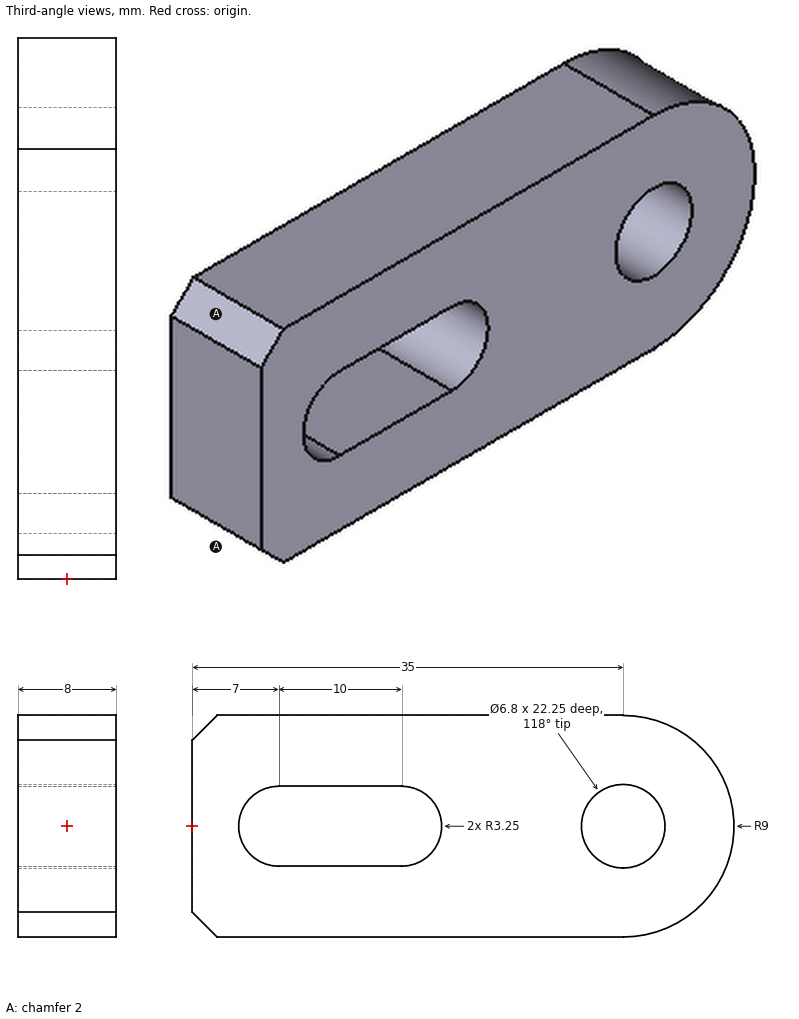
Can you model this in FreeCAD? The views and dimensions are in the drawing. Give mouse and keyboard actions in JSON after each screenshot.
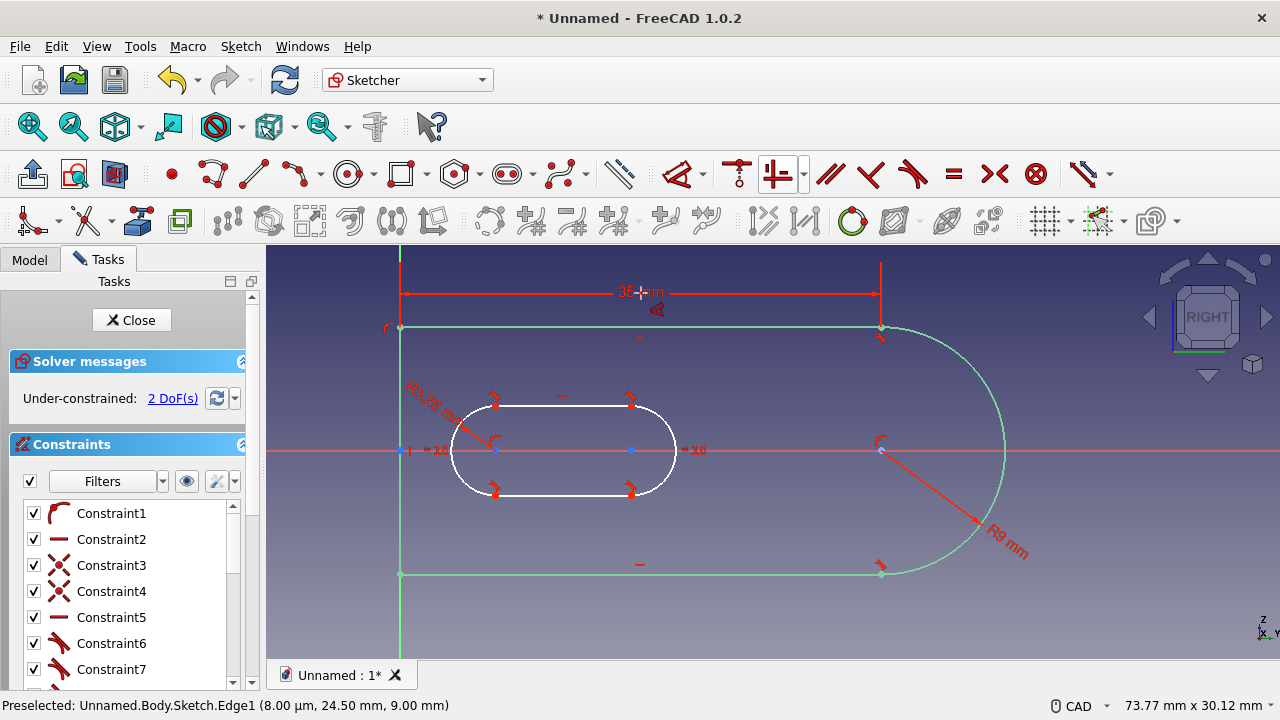
{"action": "left_click", "coordinate": [536, 406]}
{"action": "left_click", "coordinate": [564, 372]}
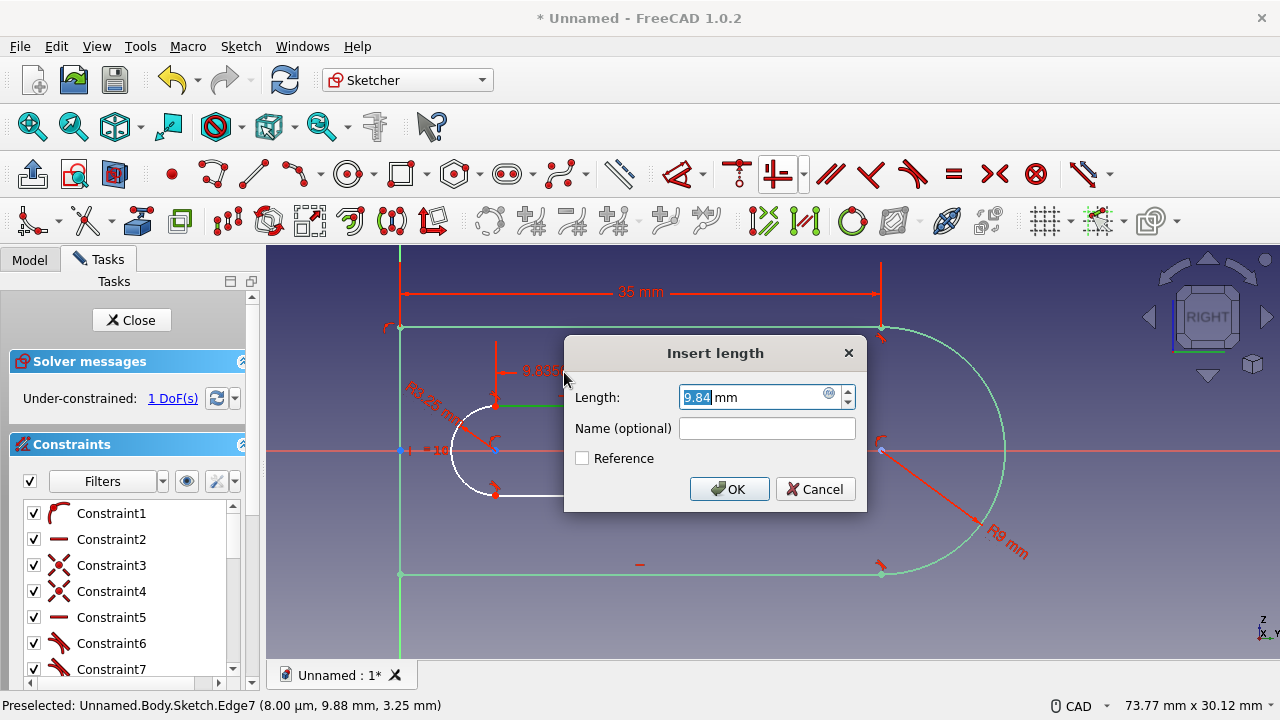
{"action": "type", "text": "10"}
{"action": "key", "text": "Return"}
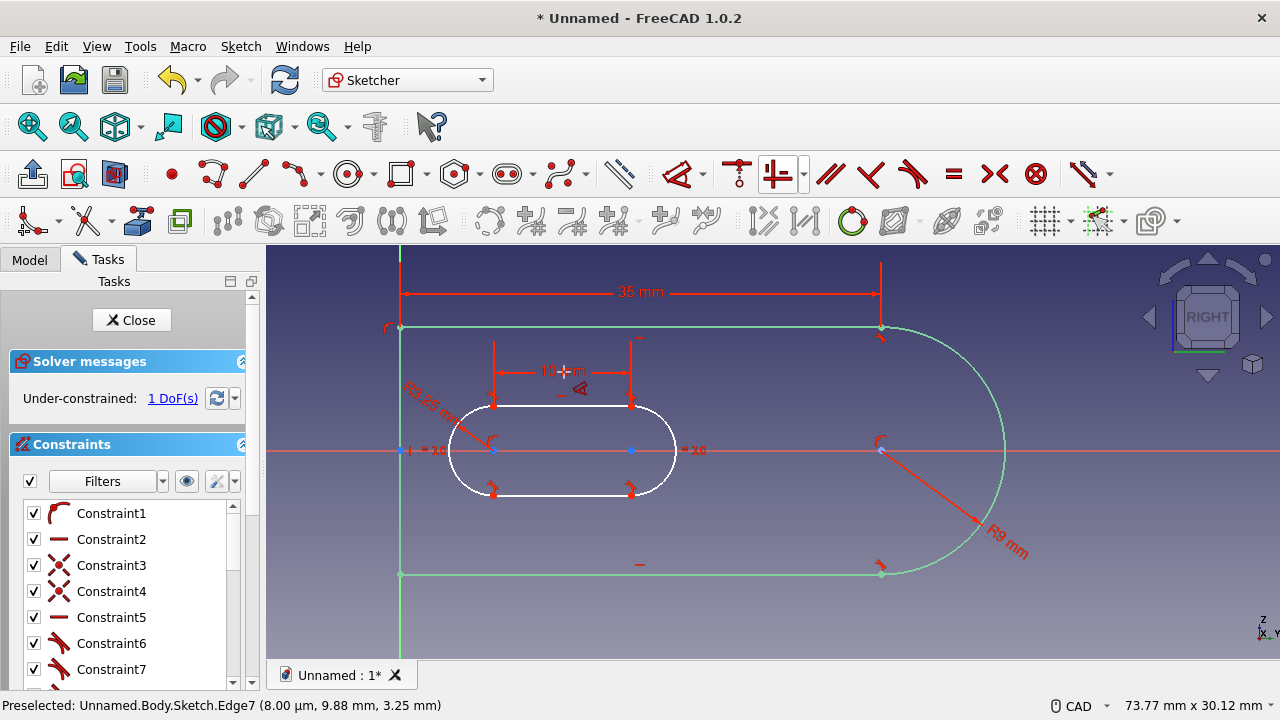
{"action": "left_click", "coordinate": [494, 406]}
{"action": "left_click", "coordinate": [447, 372]}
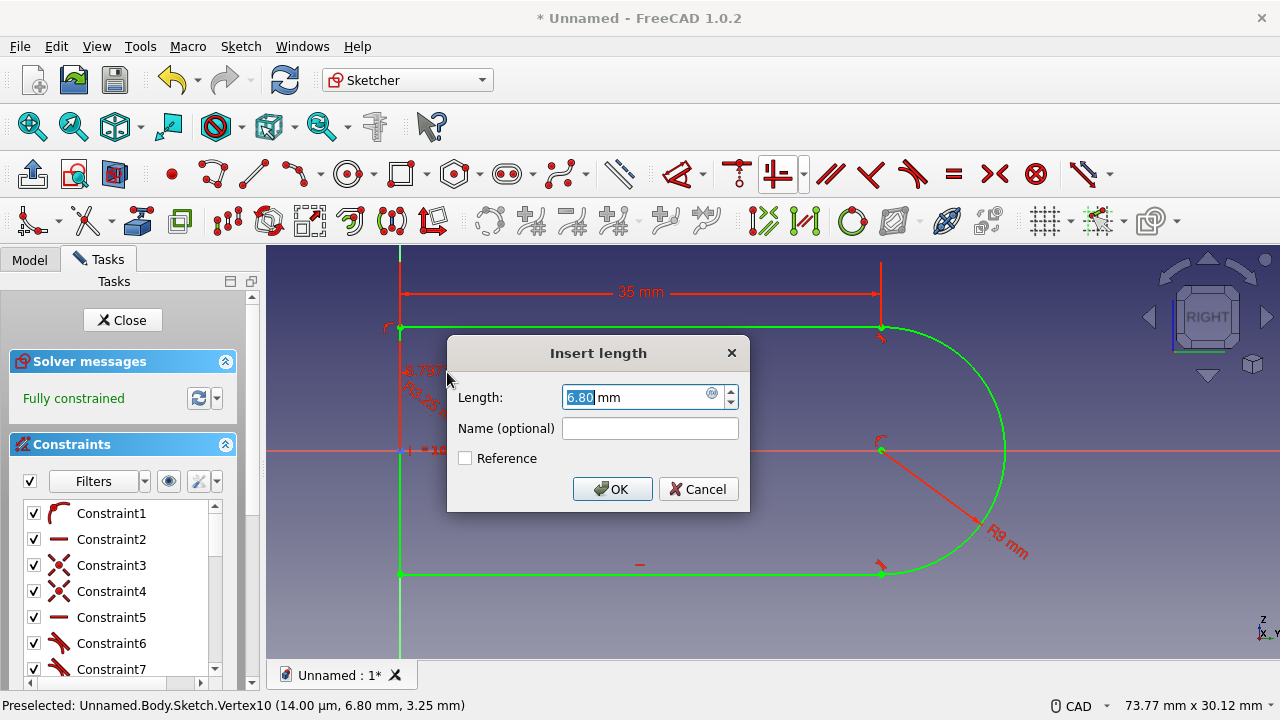
{"action": "type", "text": "7"}
{"action": "key", "text": "Return"}
{"action": "key", "text": "Escape"}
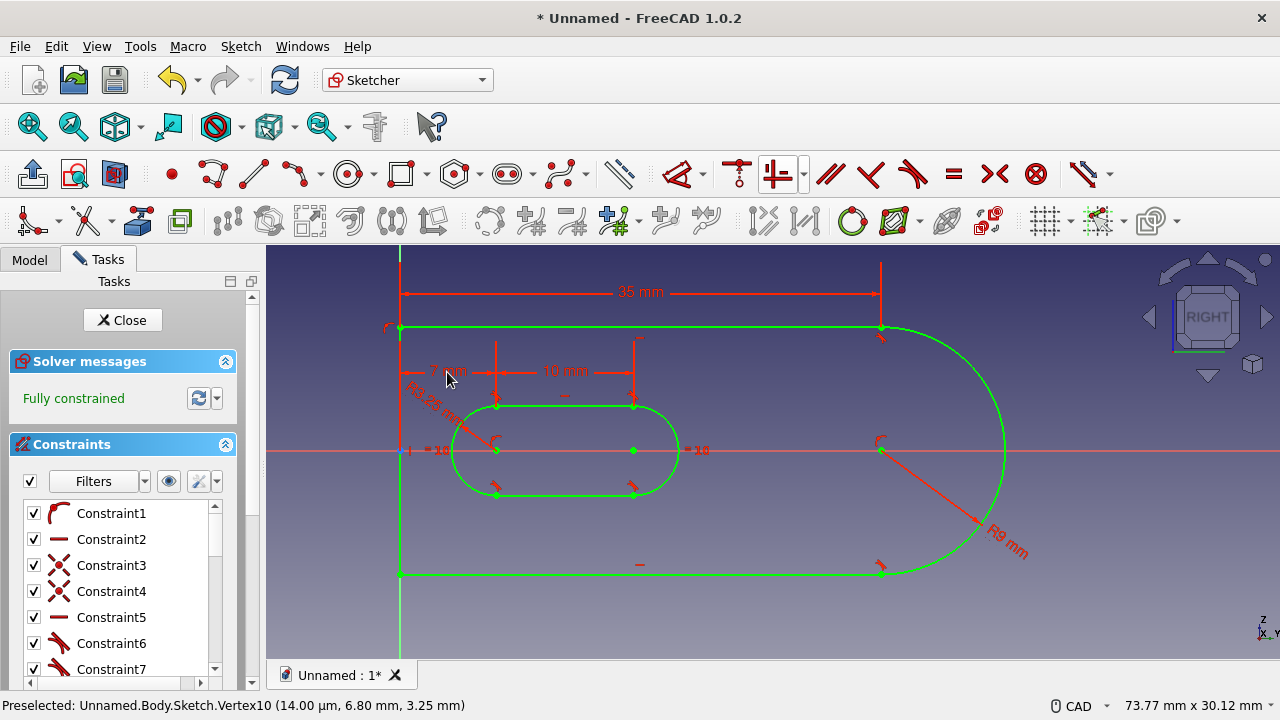
{"action": "left_click", "coordinate": [123, 320]}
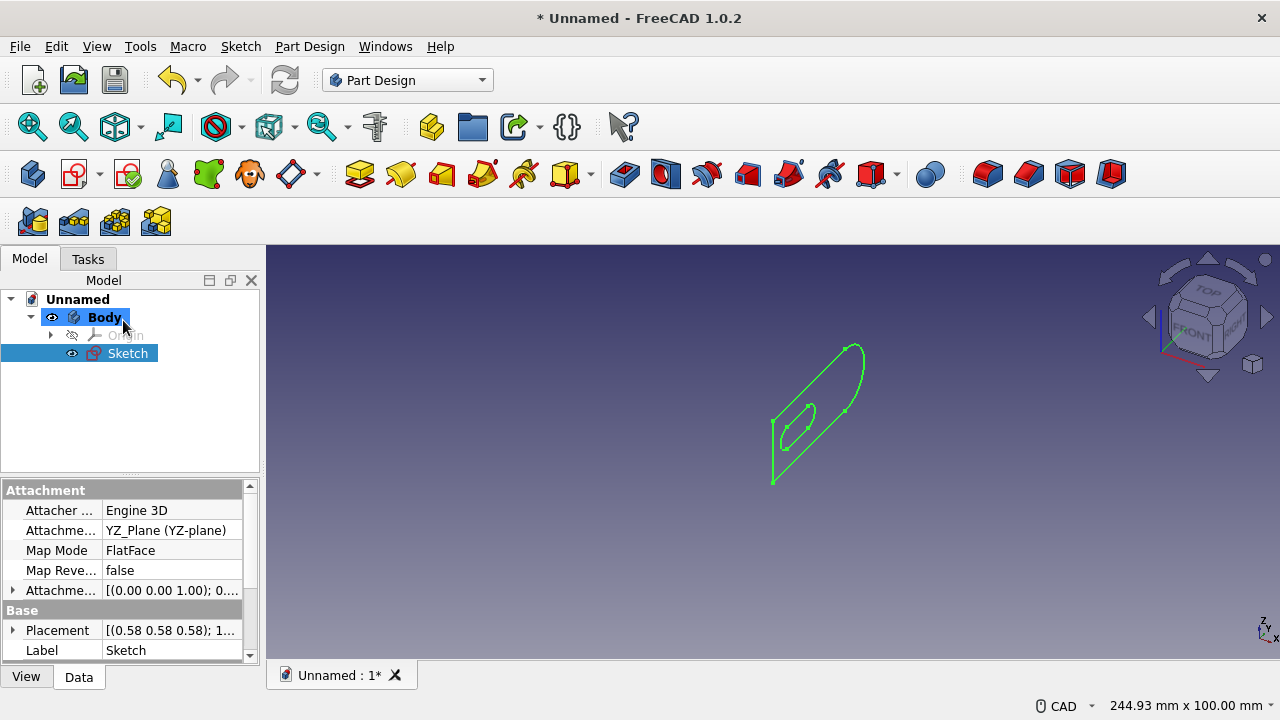
{"action": "left_click", "coordinate": [360, 174]}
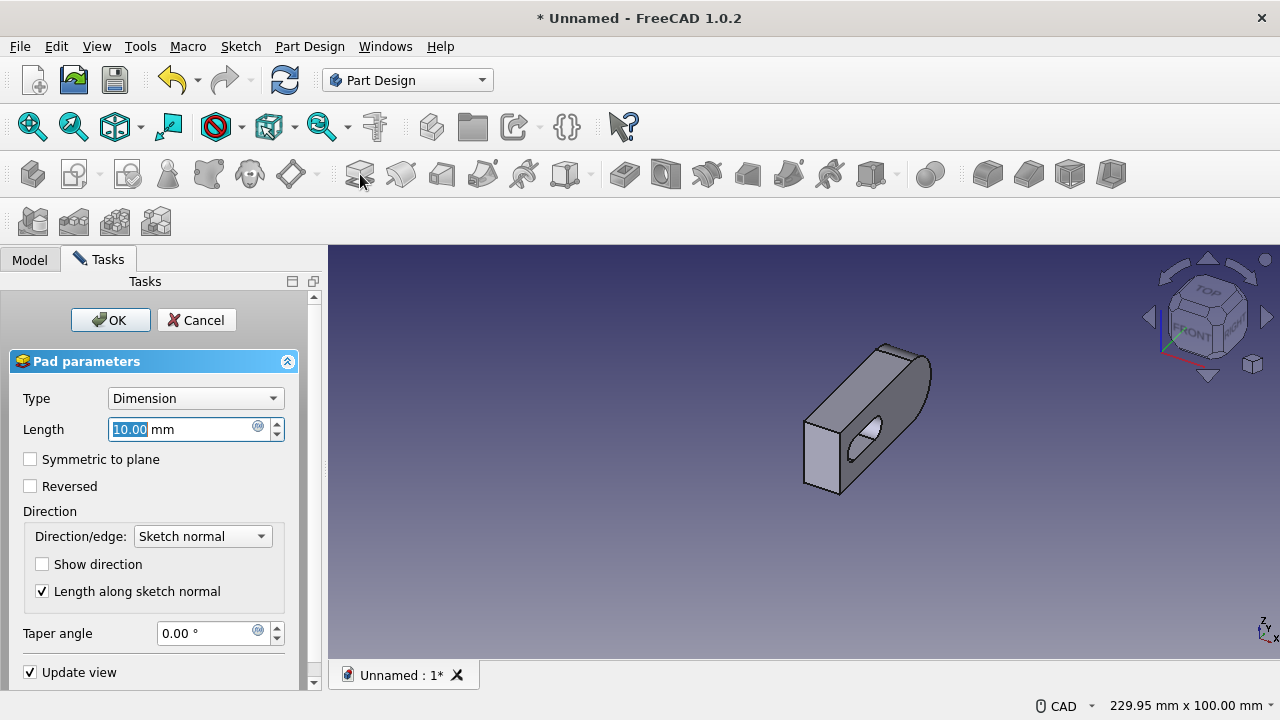
{"action": "type", "text": "8"}
{"action": "key", "text": "Tab"}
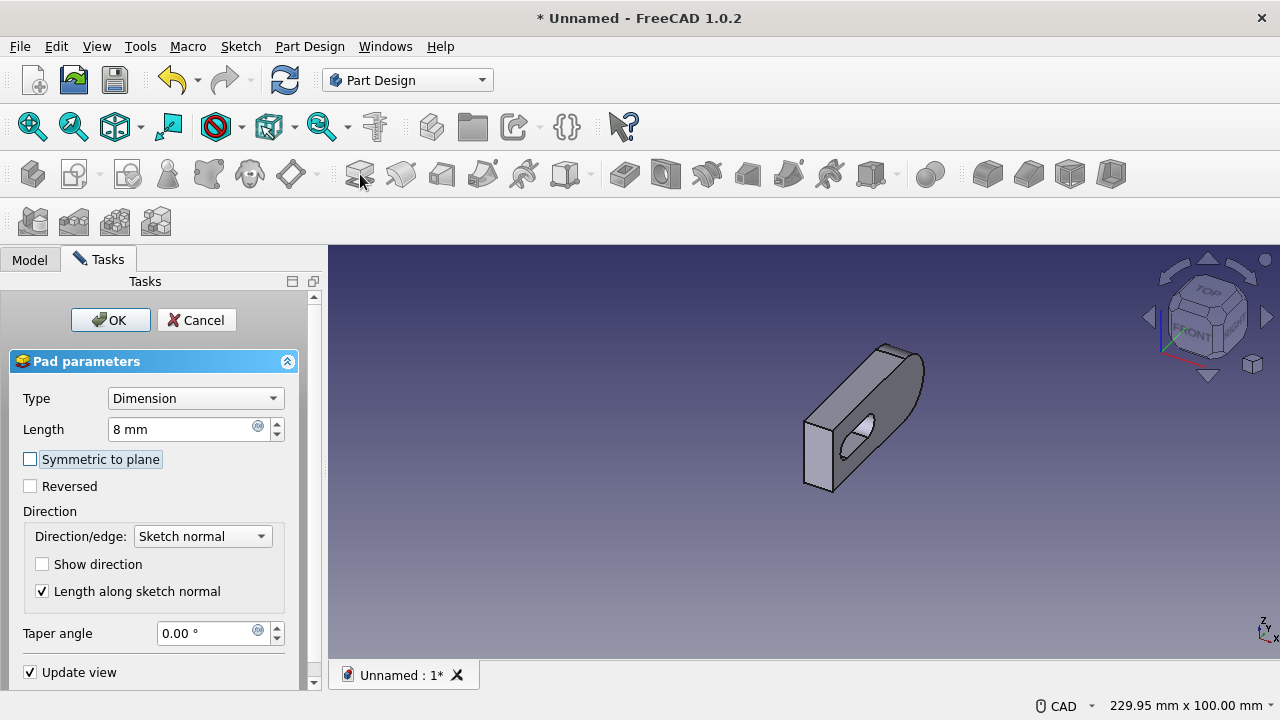
{"action": "left_click", "coordinate": [31, 459]}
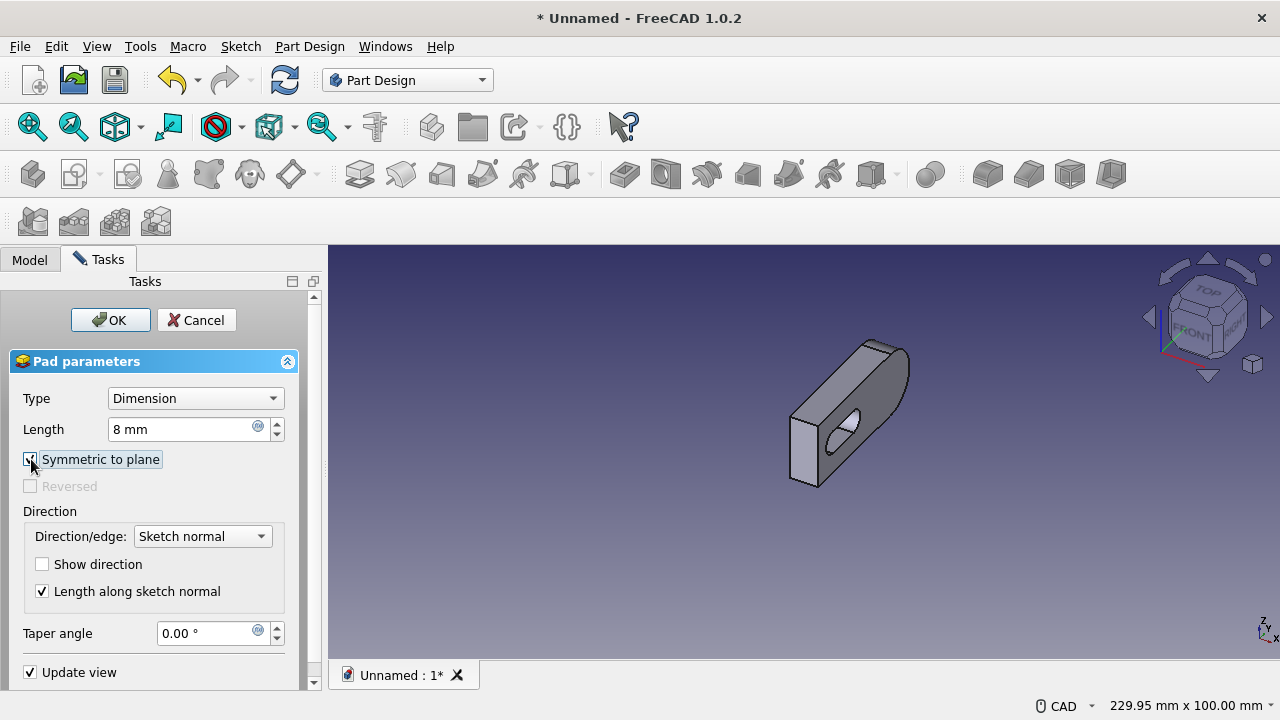
{"action": "left_click", "coordinate": [111, 320]}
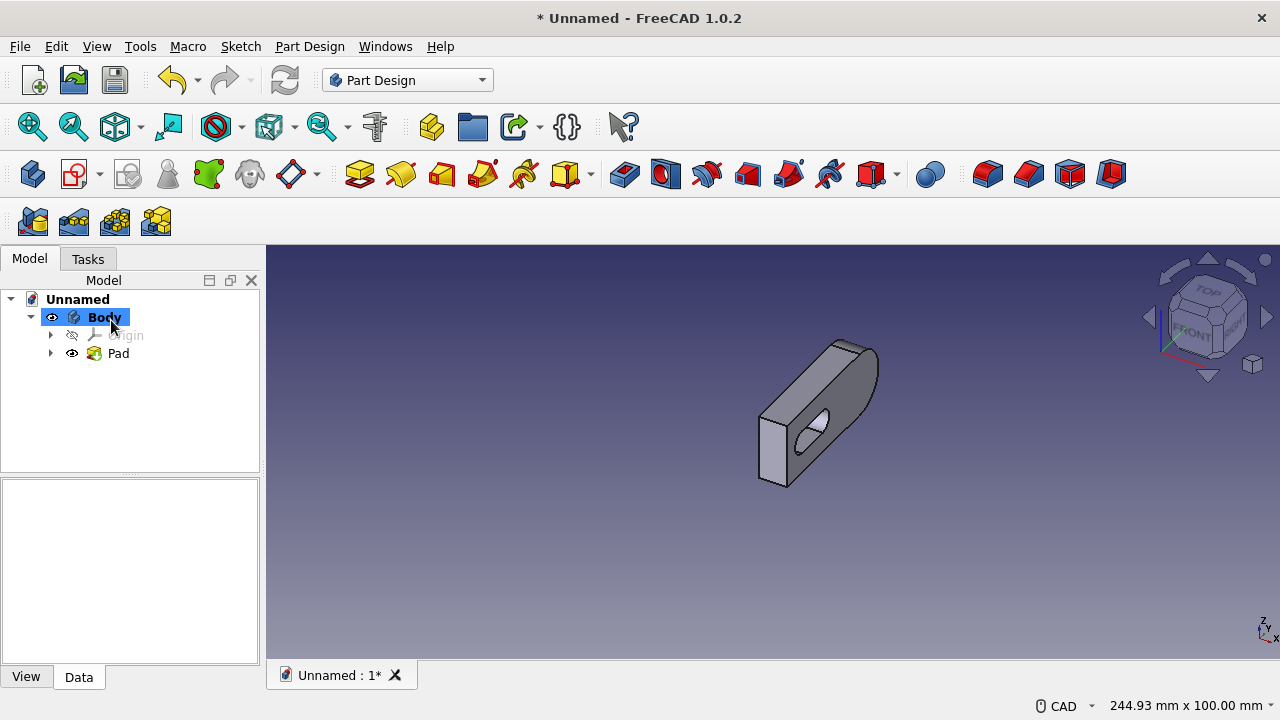
{"action": "left_click", "coordinate": [33, 128]}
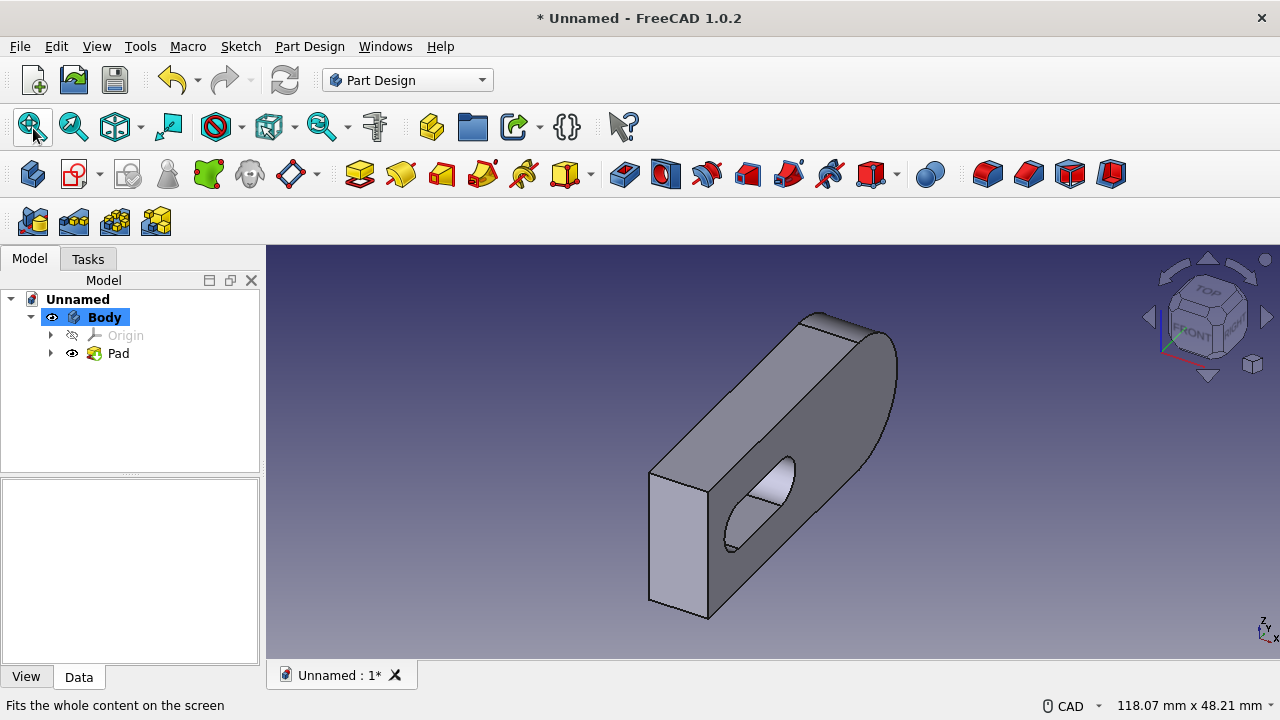
{"action": "key", "text": "6"}